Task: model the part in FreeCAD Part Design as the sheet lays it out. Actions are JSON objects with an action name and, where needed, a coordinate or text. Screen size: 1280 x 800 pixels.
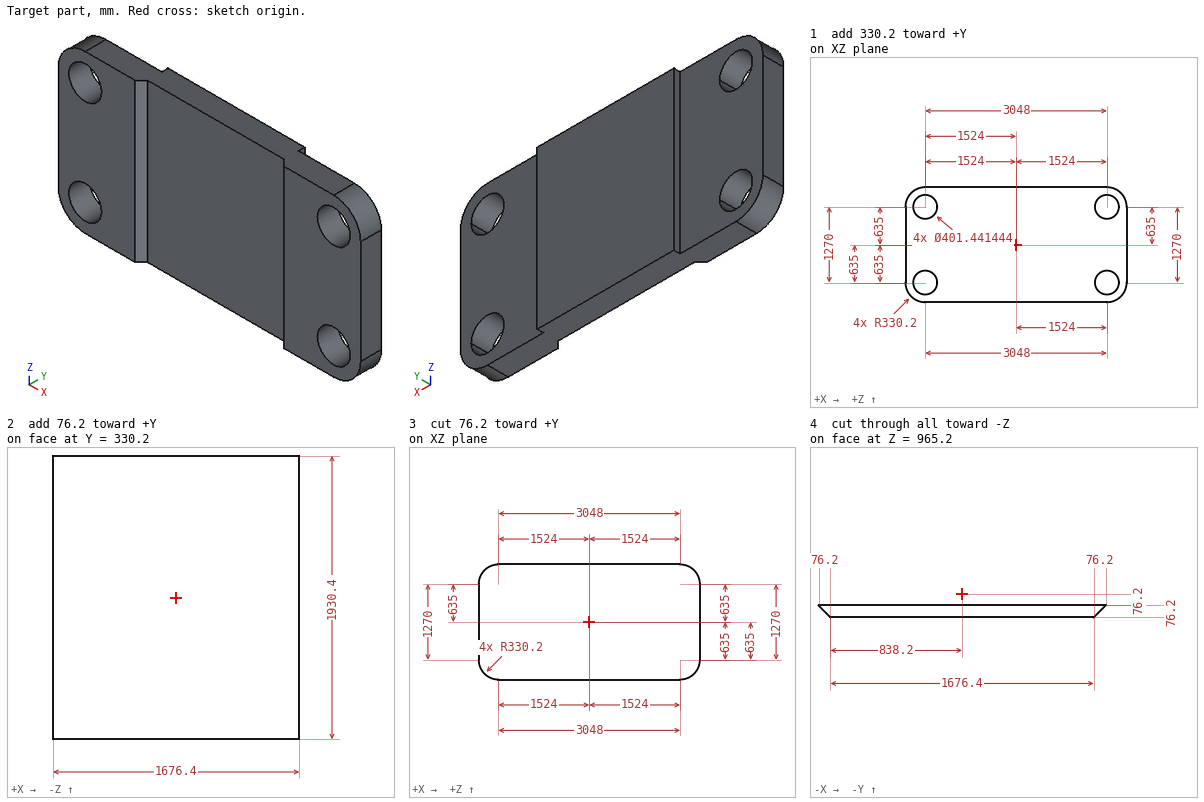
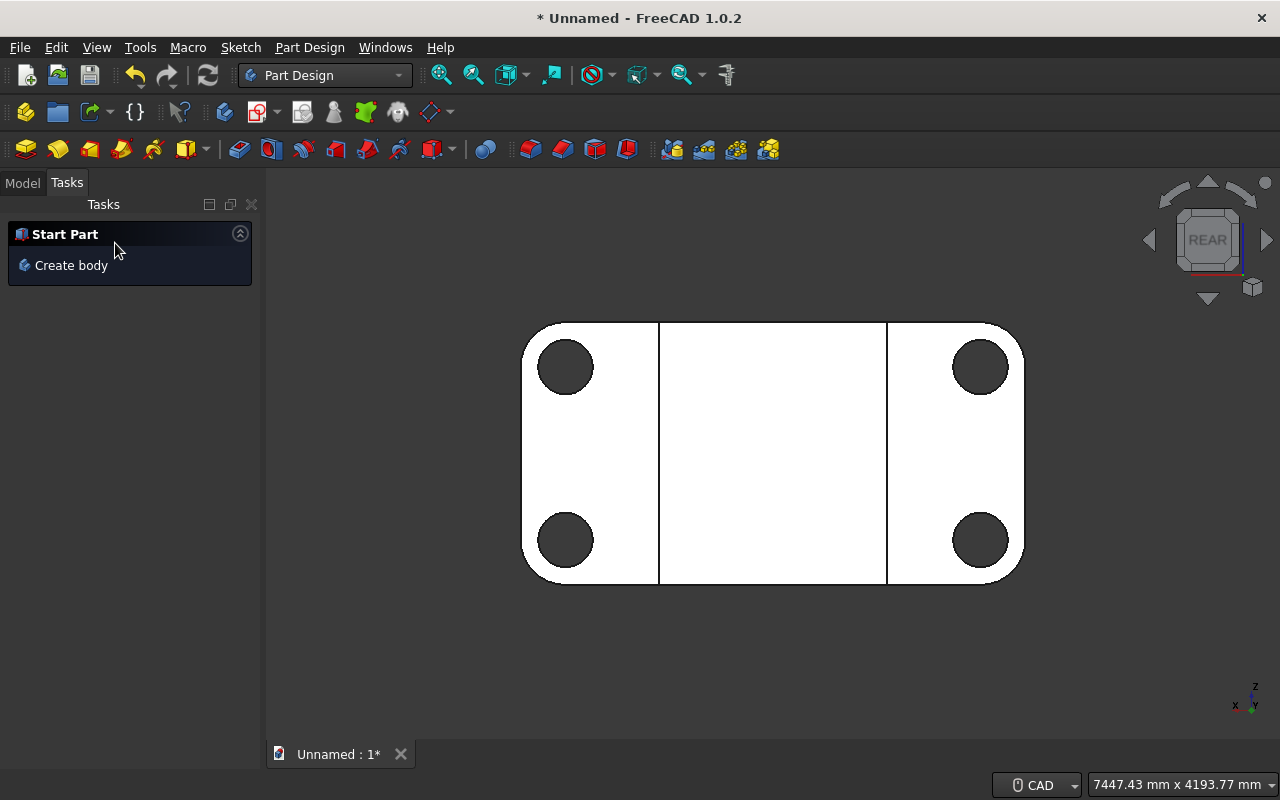
{"action": "left_click", "coordinate": [258, 112]}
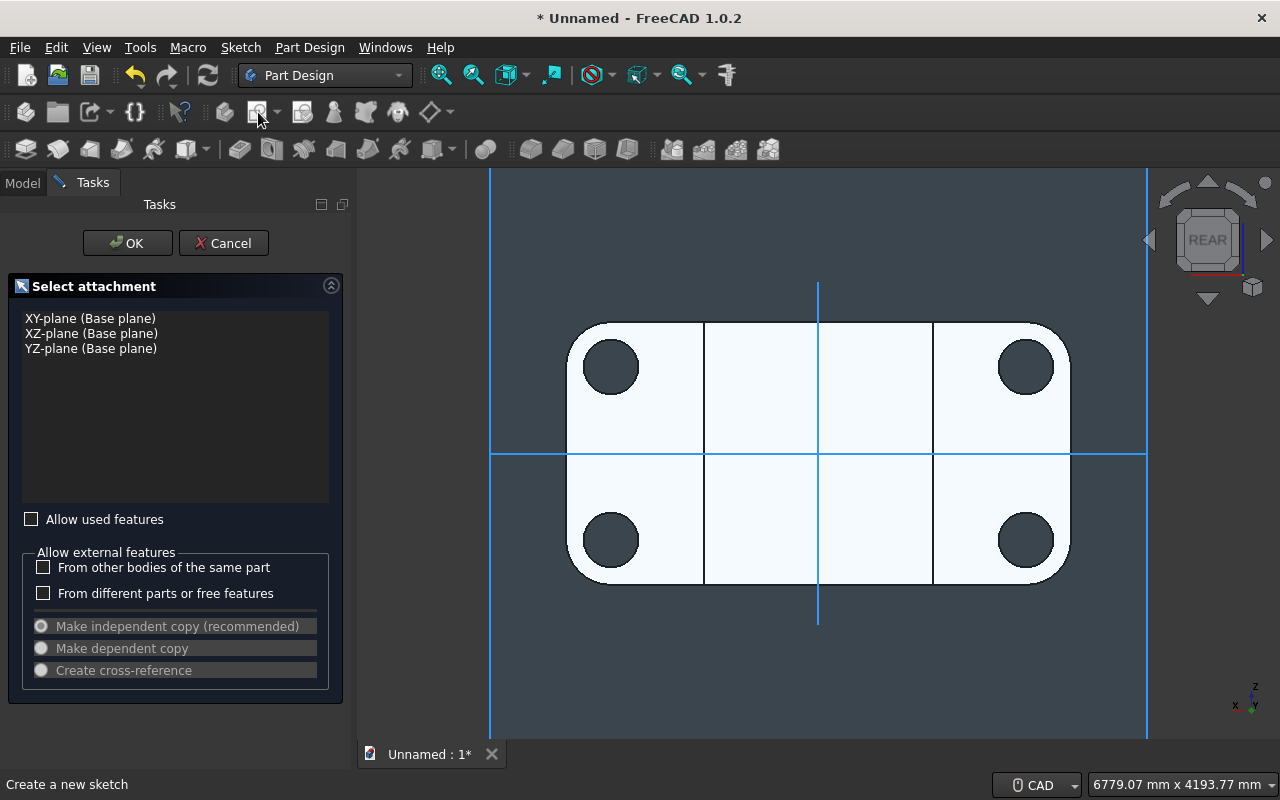
{"action": "left_click", "coordinate": [82, 334]}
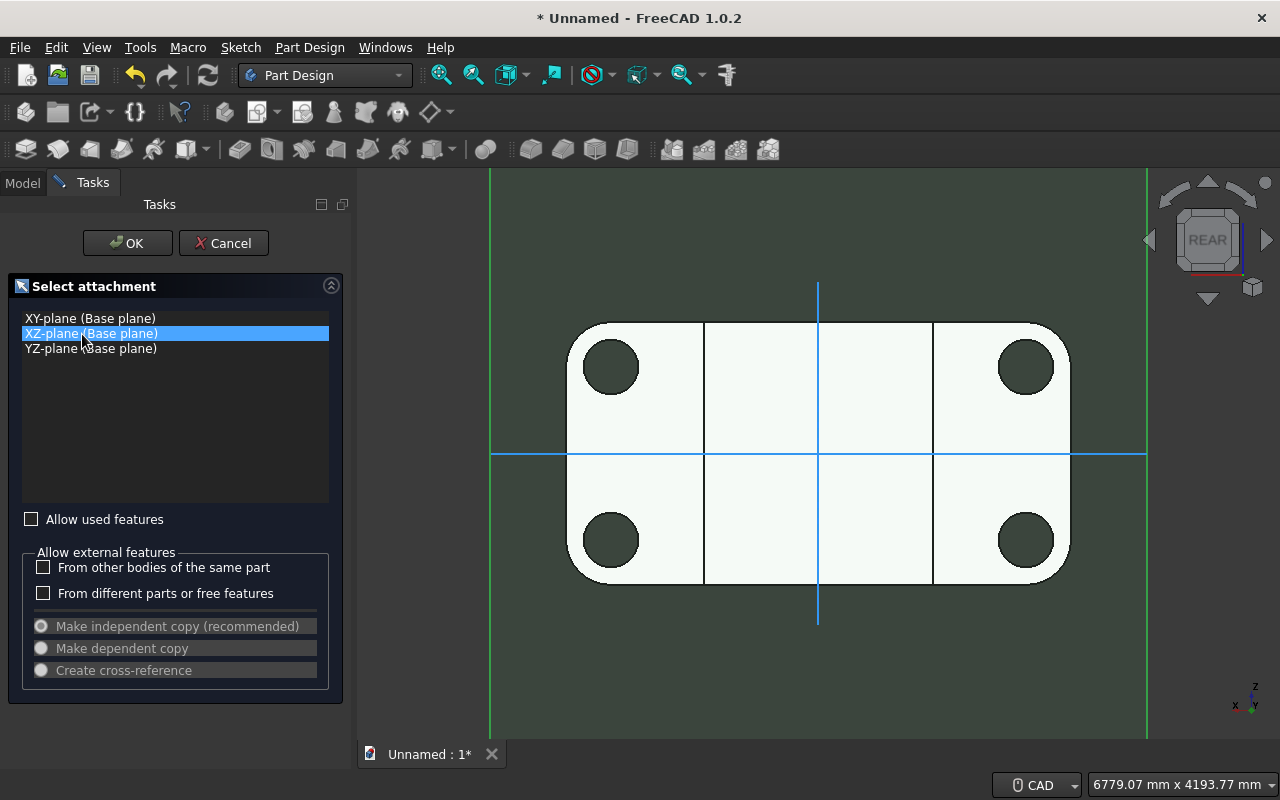
{"action": "left_click", "coordinate": [128, 243]}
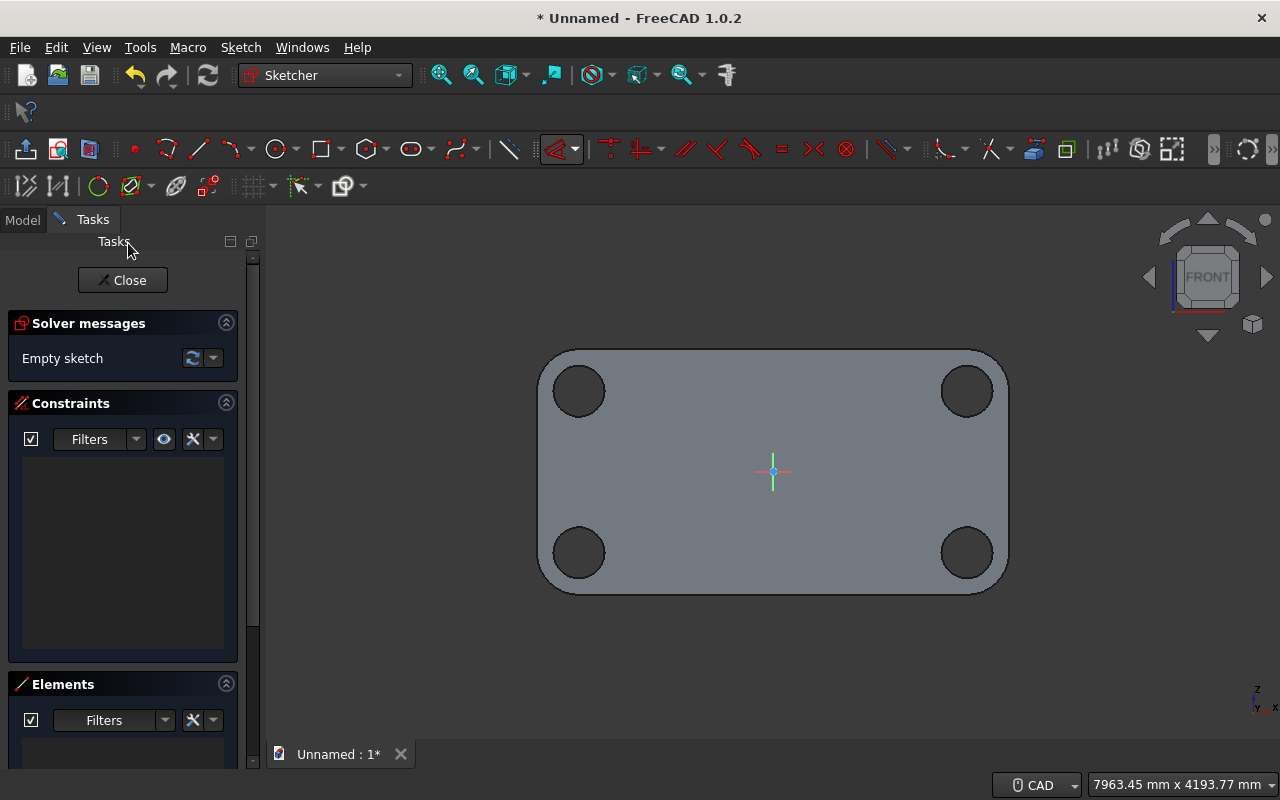
{"action": "left_click", "coordinate": [200, 150]}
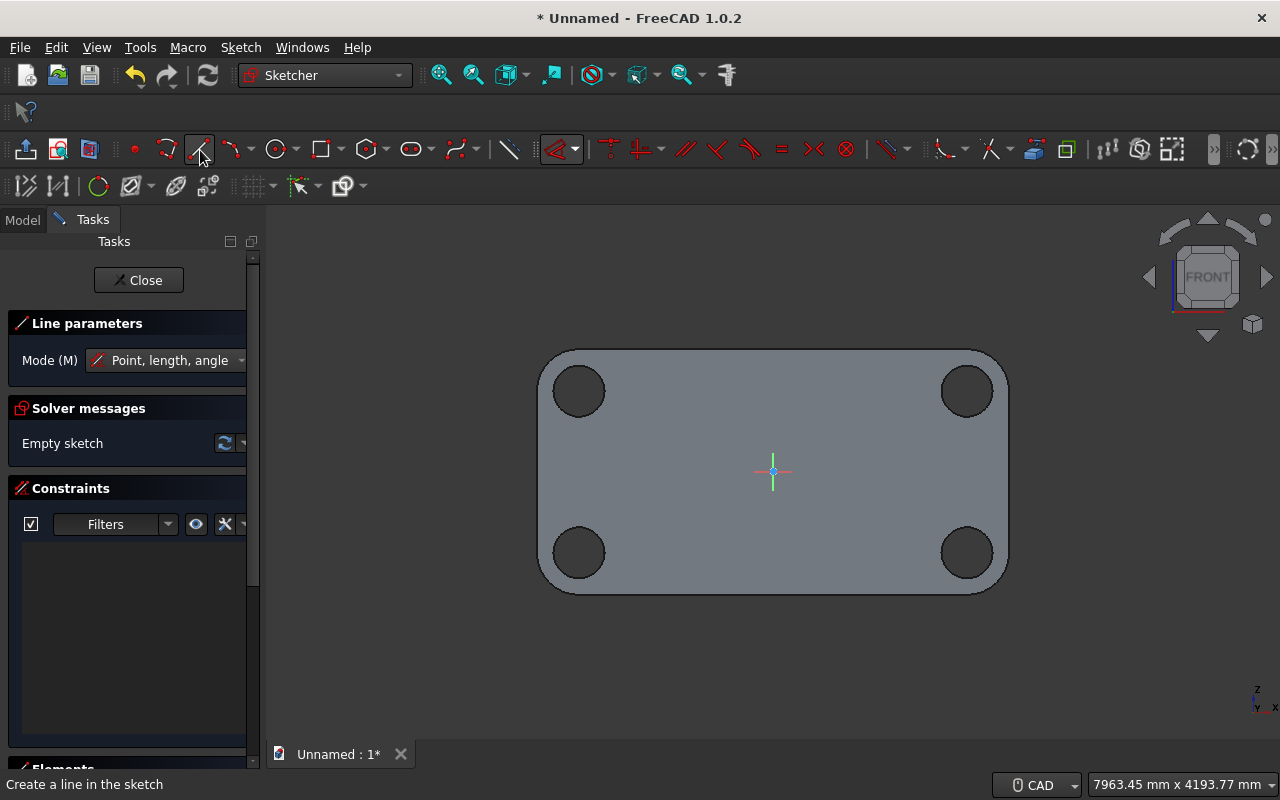
{"action": "left_click", "coordinate": [579, 595]}
{"action": "left_click", "coordinate": [967, 595]}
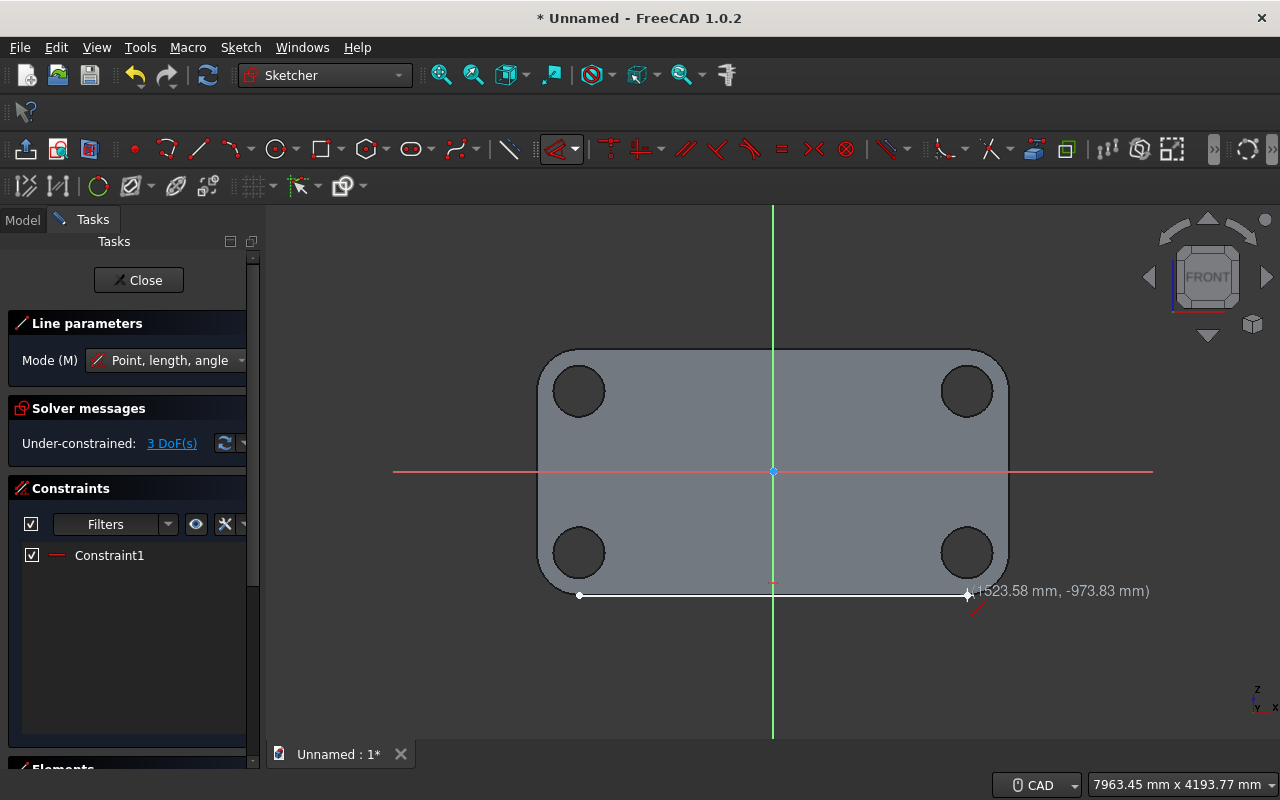
{"action": "left_click", "coordinate": [1009, 553]}
{"action": "left_click", "coordinate": [1009, 391]}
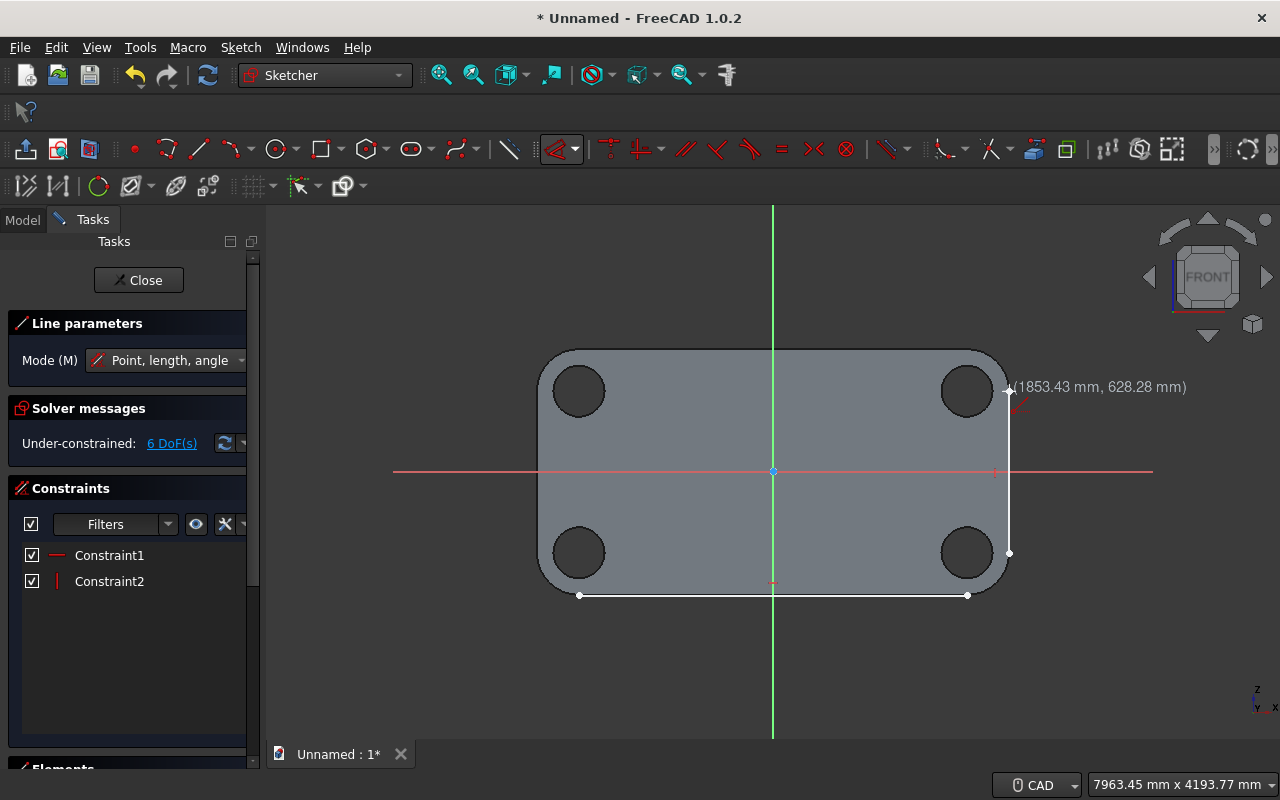
{"action": "left_click", "coordinate": [967, 349]}
{"action": "left_click", "coordinate": [579, 349]}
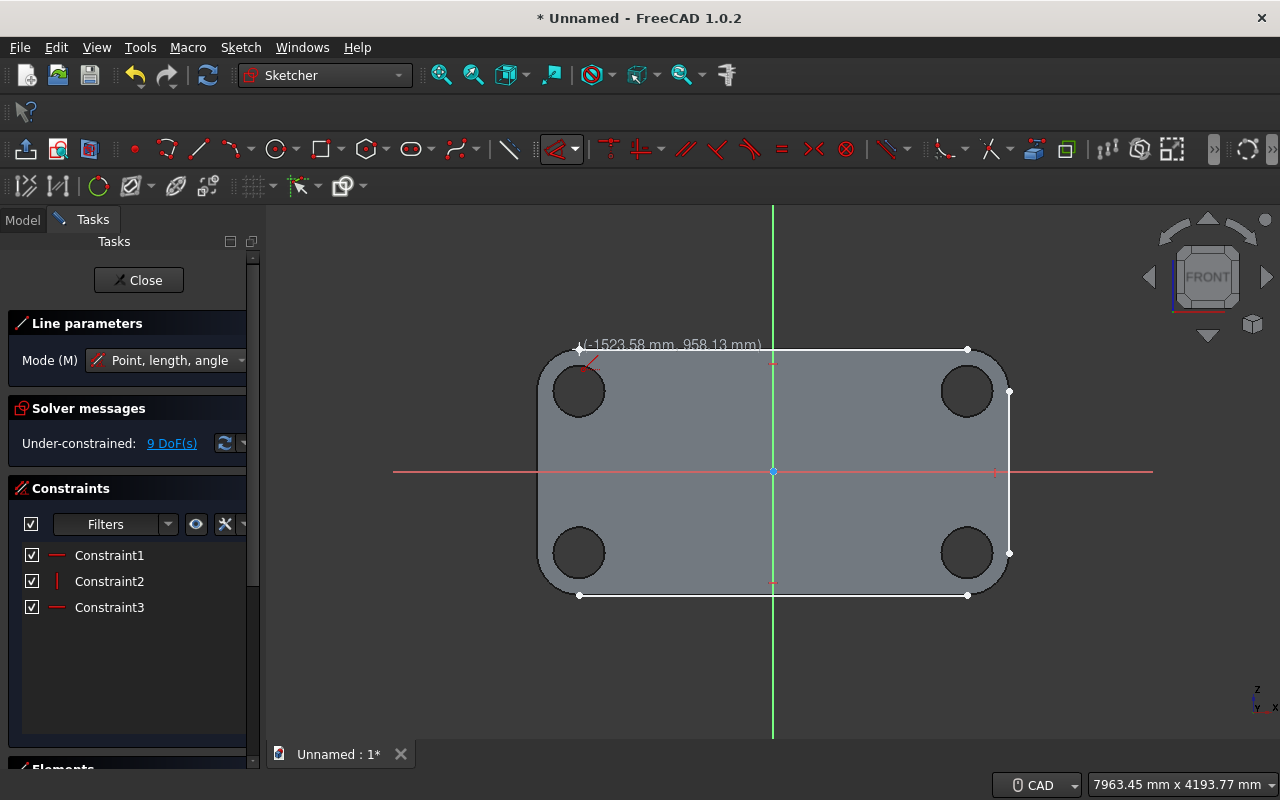
{"action": "left_click", "coordinate": [537, 391]}
{"action": "left_click", "coordinate": [537, 553]}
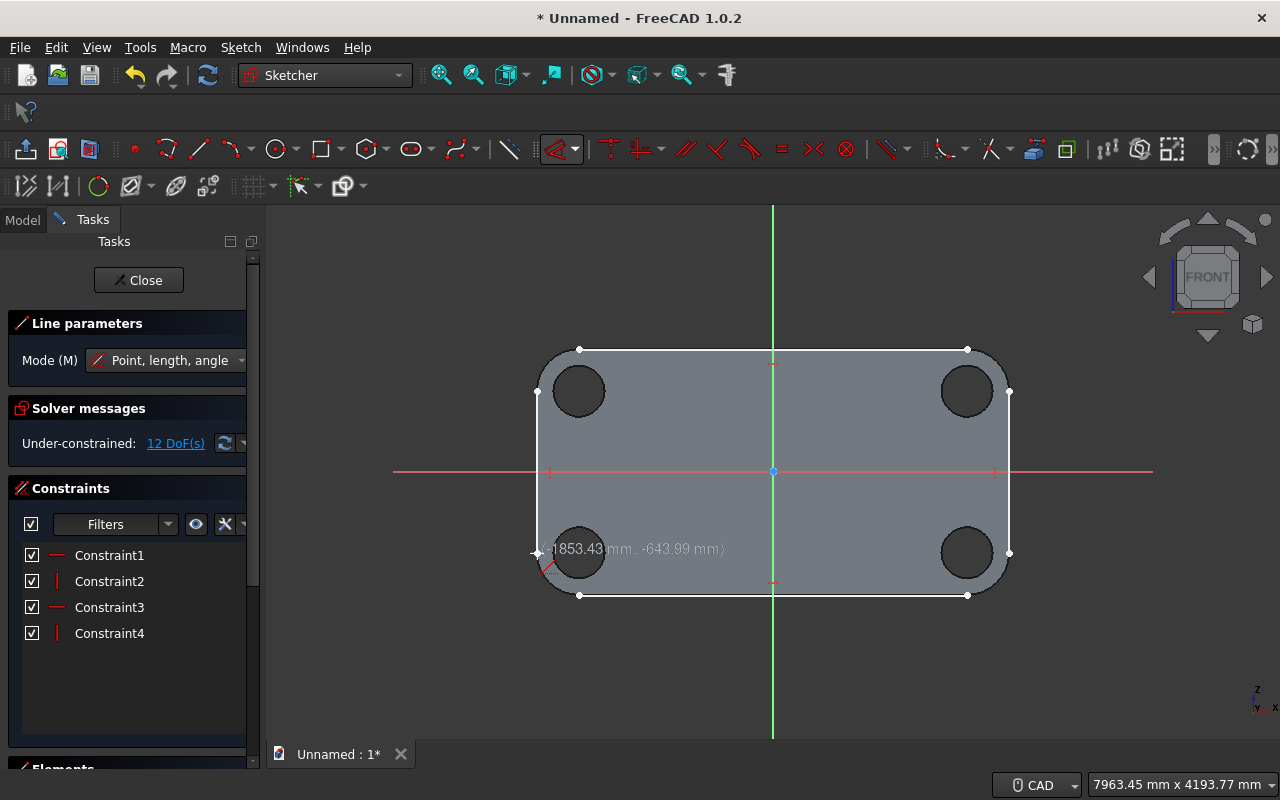
{"action": "key", "text": "g 3 a"}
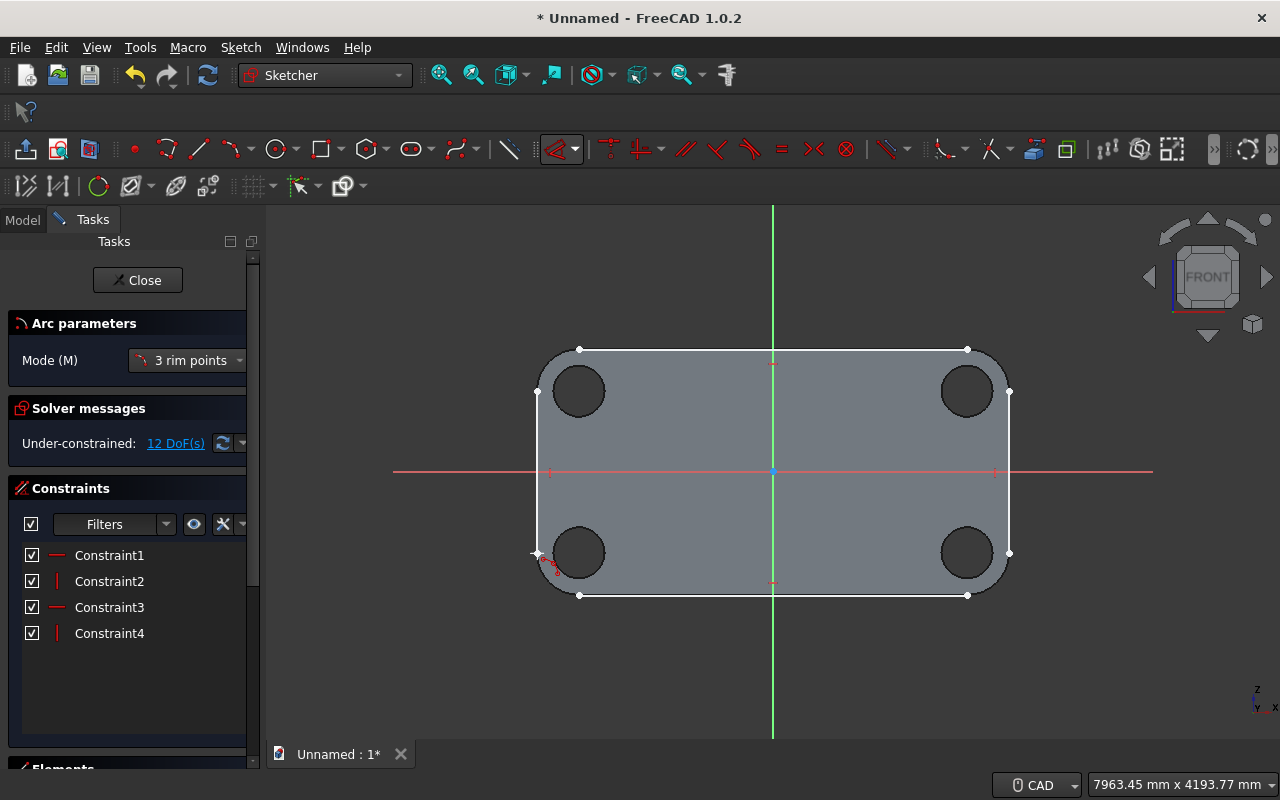
{"action": "left_click", "coordinate": [967, 596]}
{"action": "left_click", "coordinate": [1009, 554]}